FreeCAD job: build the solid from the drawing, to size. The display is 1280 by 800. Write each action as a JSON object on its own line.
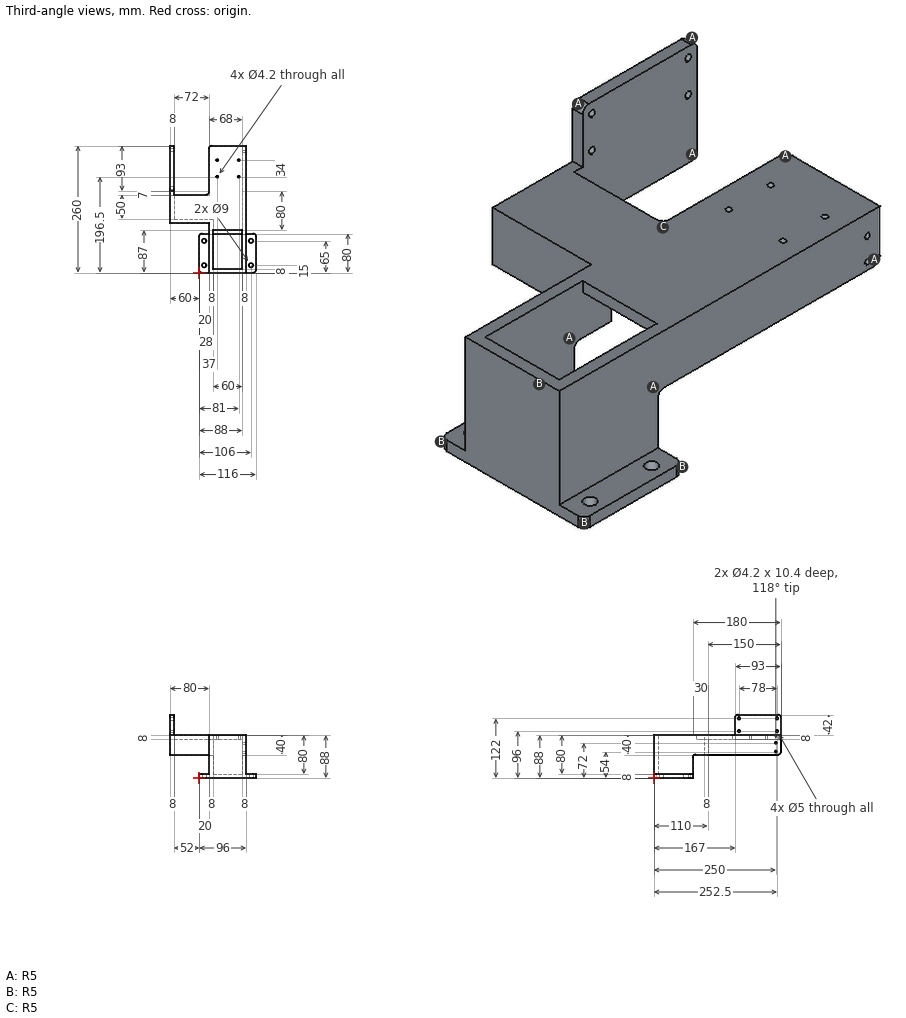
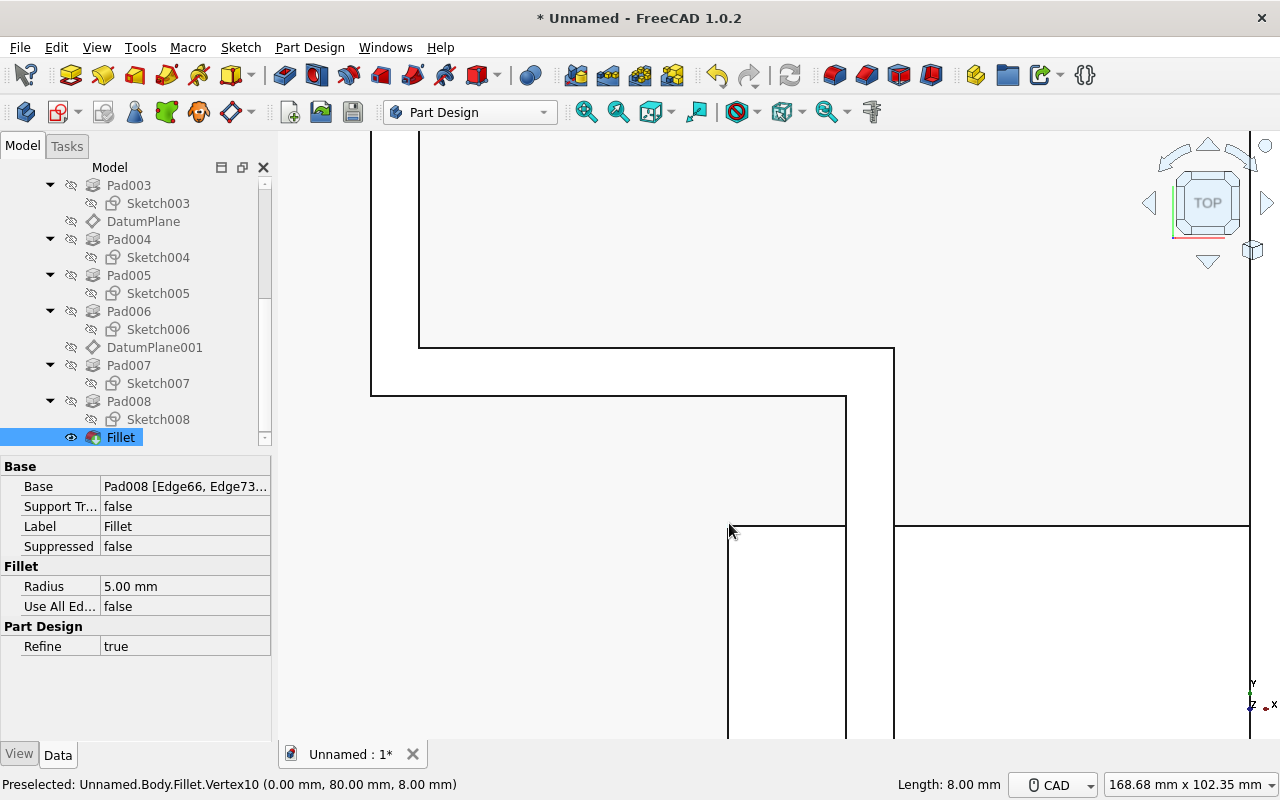
{"action": "left_click", "coordinate": [588, 112]}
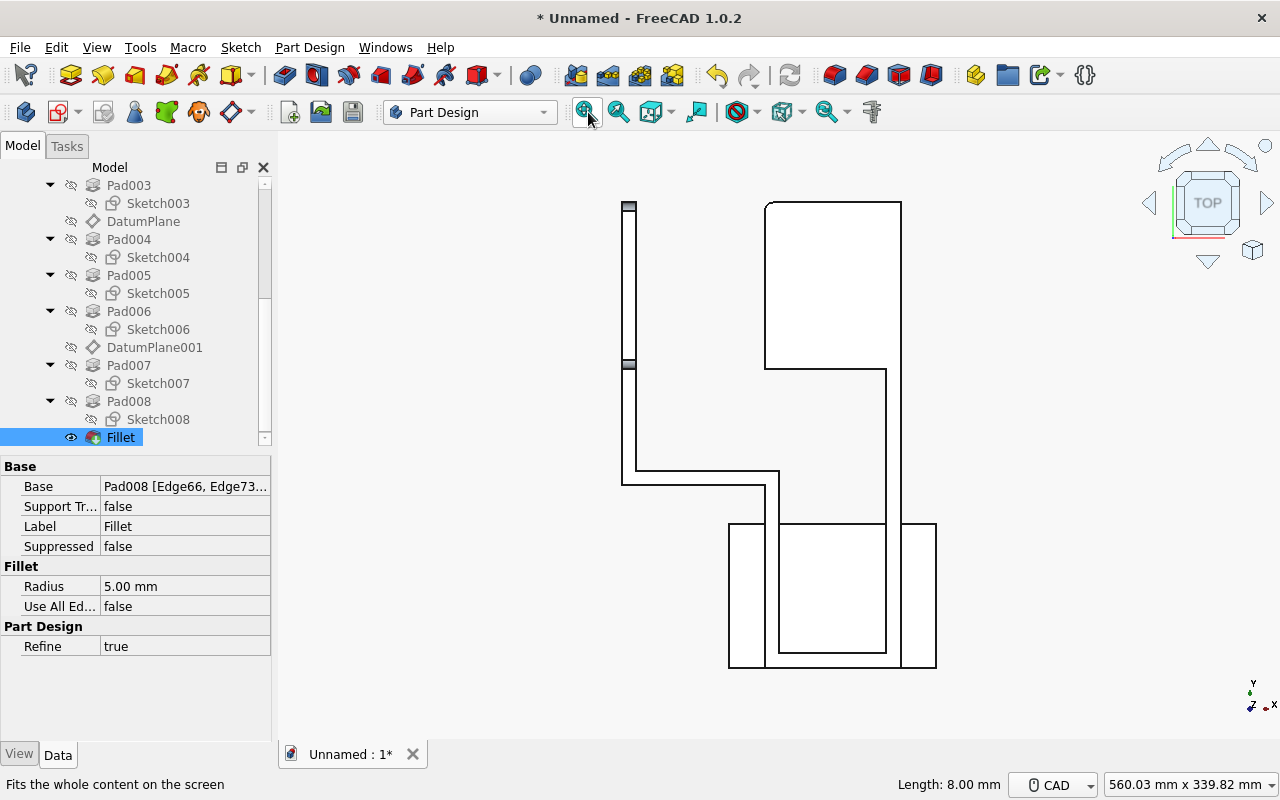
{"action": "key", "text": "0"}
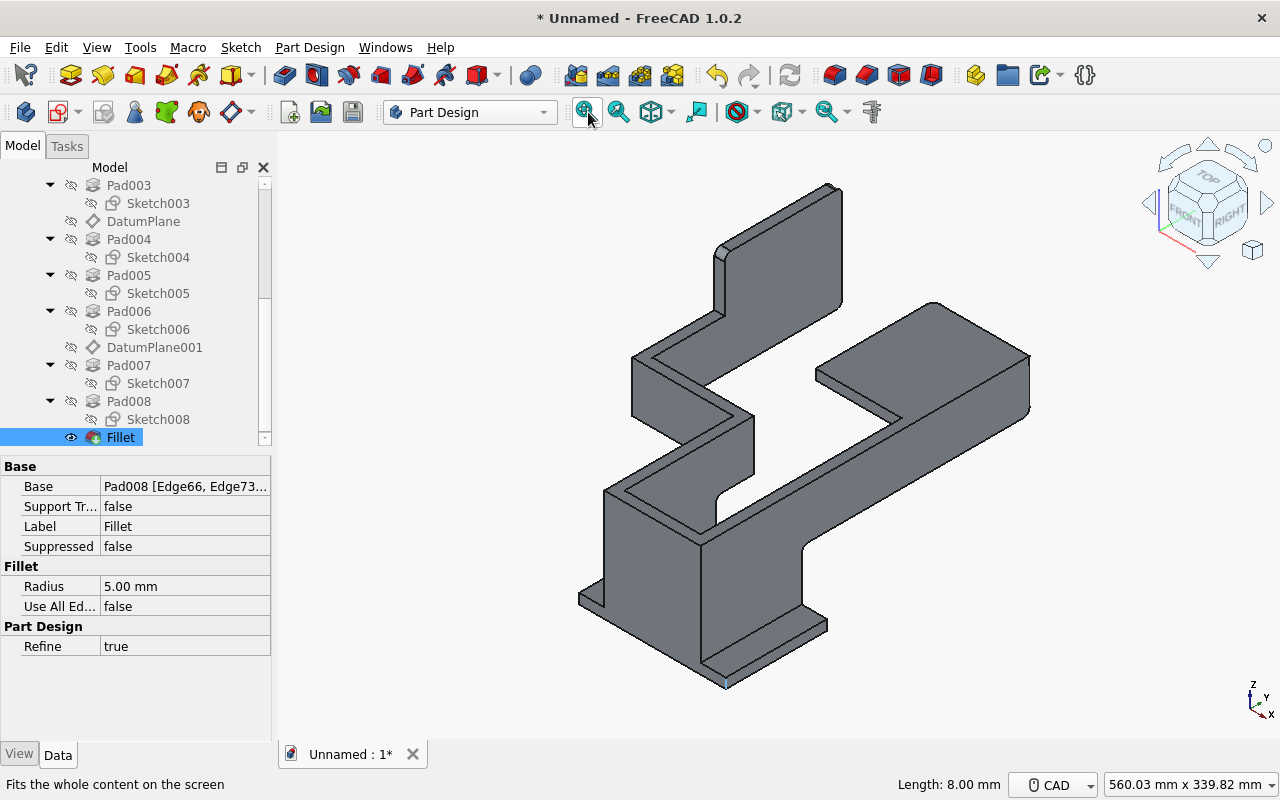
{"action": "scroll", "coordinate": [680, 539], "scroll_direction": "up", "scroll_amount": 6}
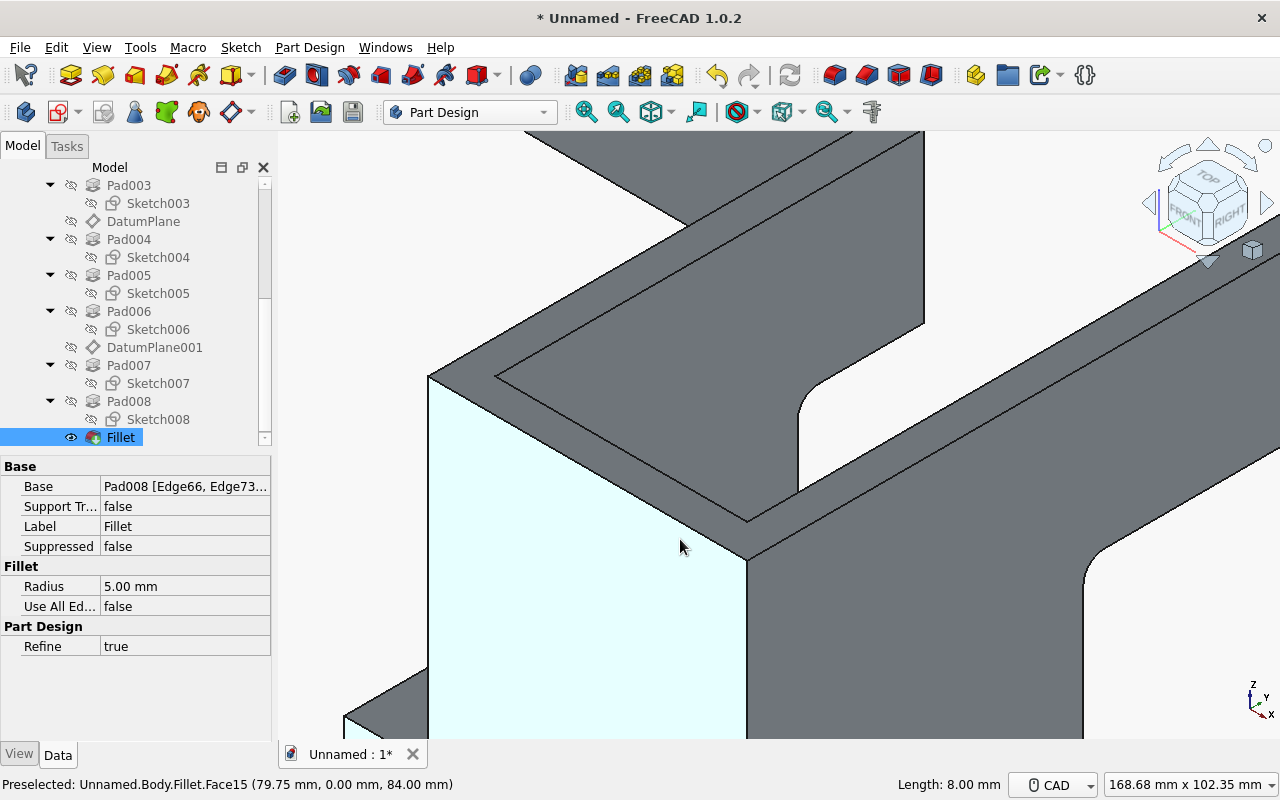
{"action": "left_click", "coordinate": [588, 112]}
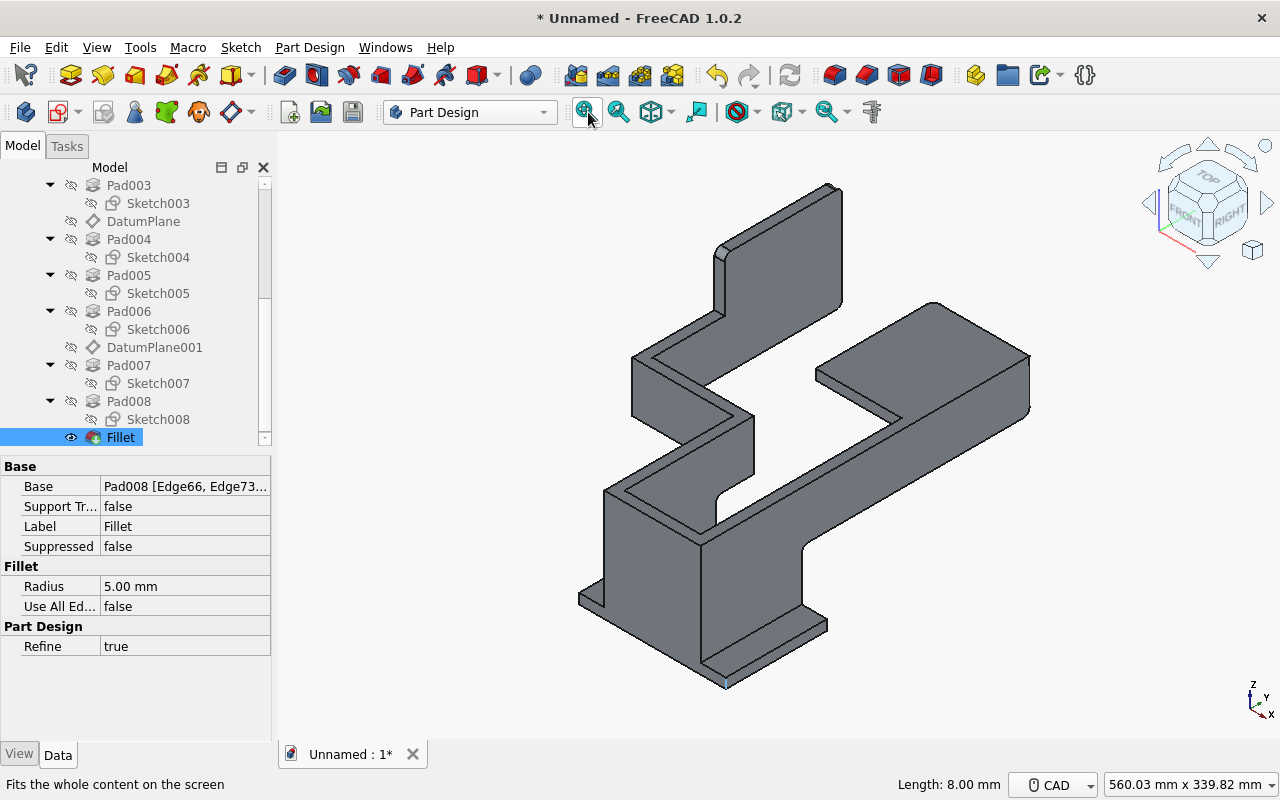
{"action": "key", "text": "1"}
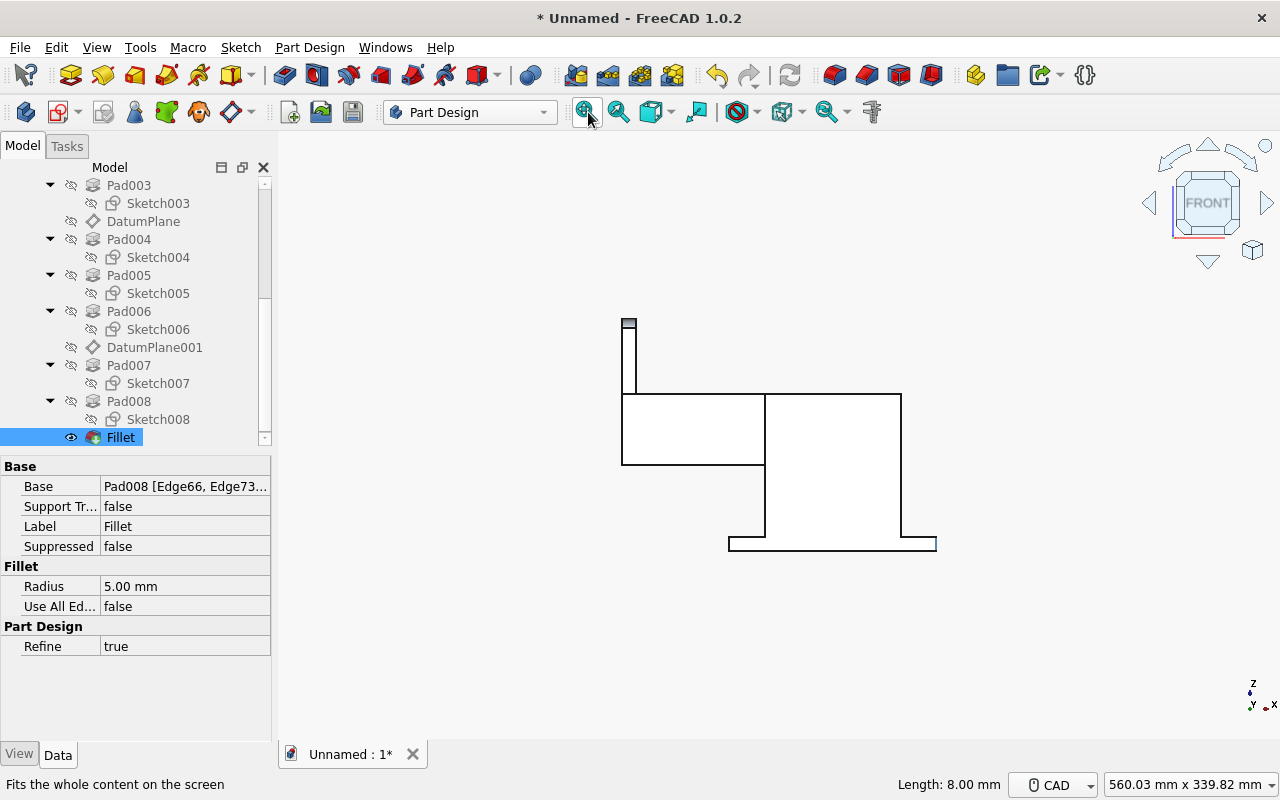
{"action": "left_click", "coordinate": [588, 112]}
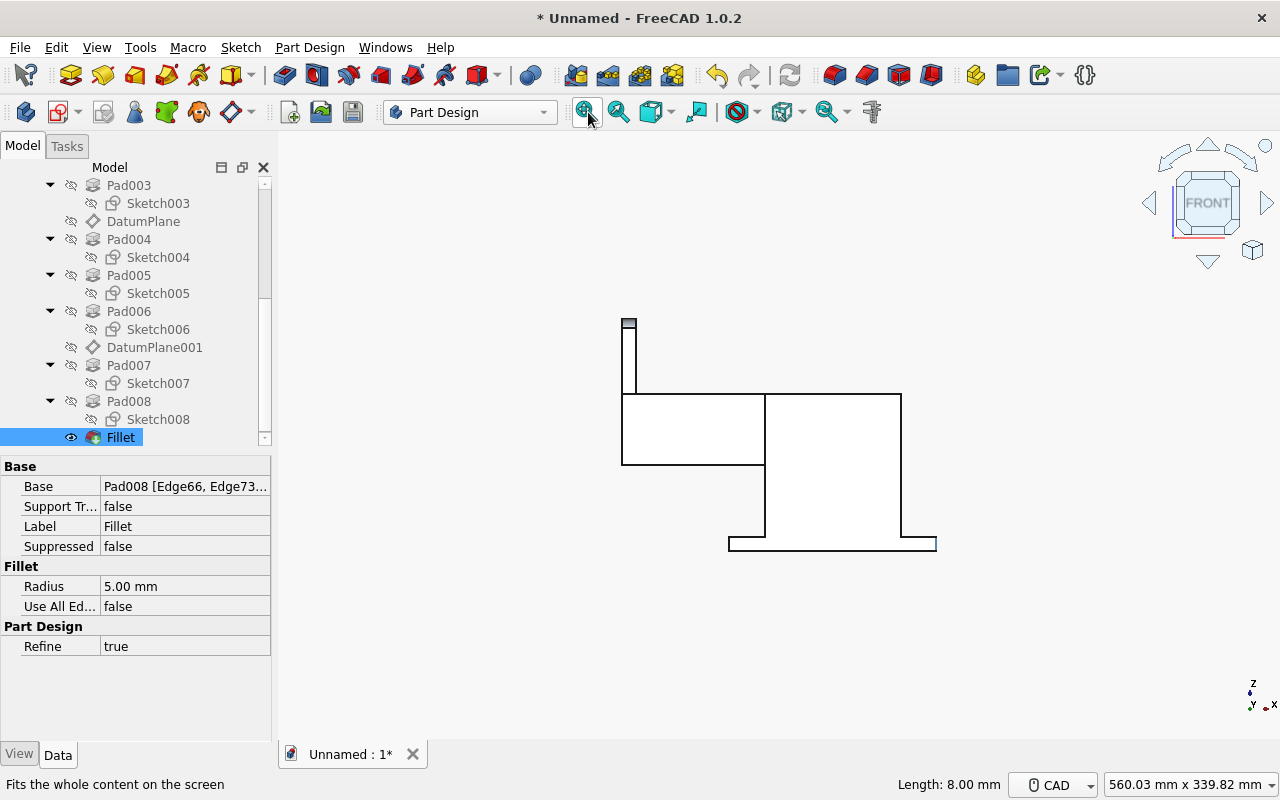
{"action": "left_click", "coordinate": [729, 543], "text": "ctrl"}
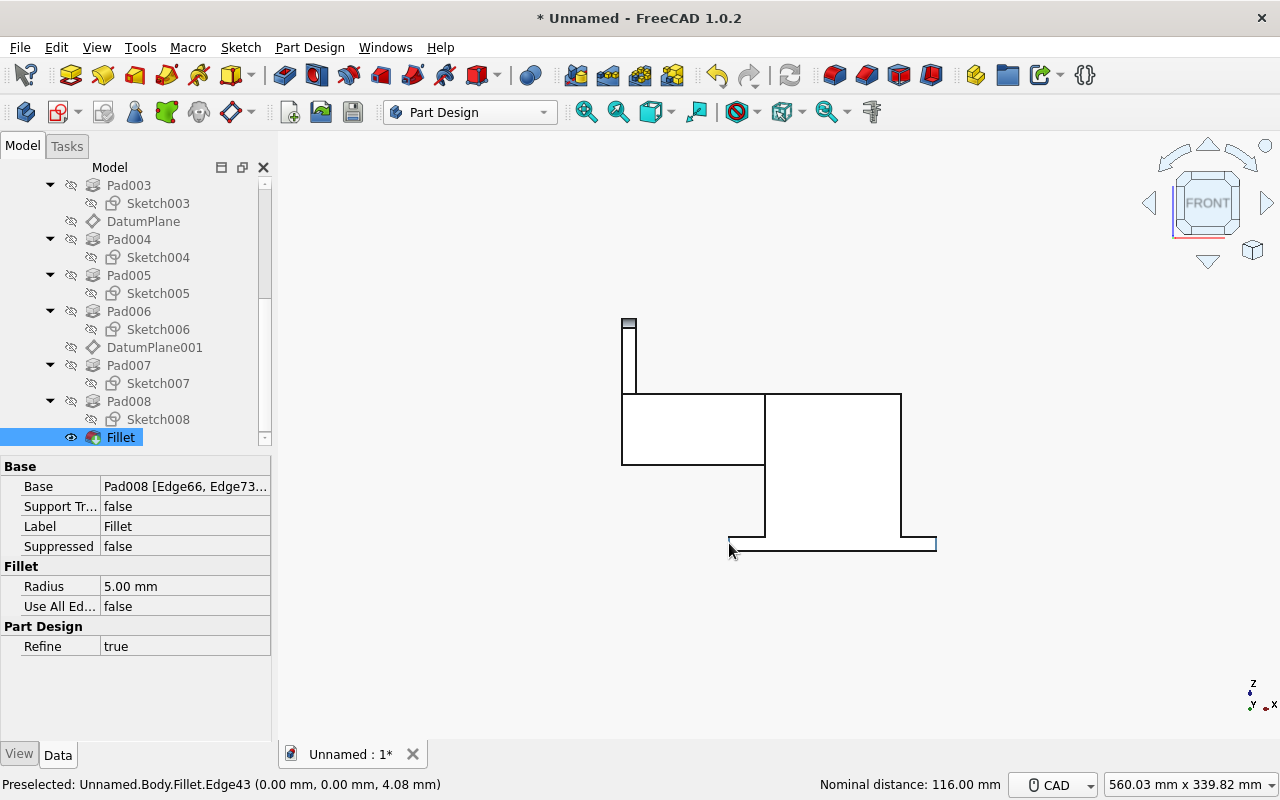
{"action": "scroll", "coordinate": [729, 543], "scroll_direction": "up", "scroll_amount": 6}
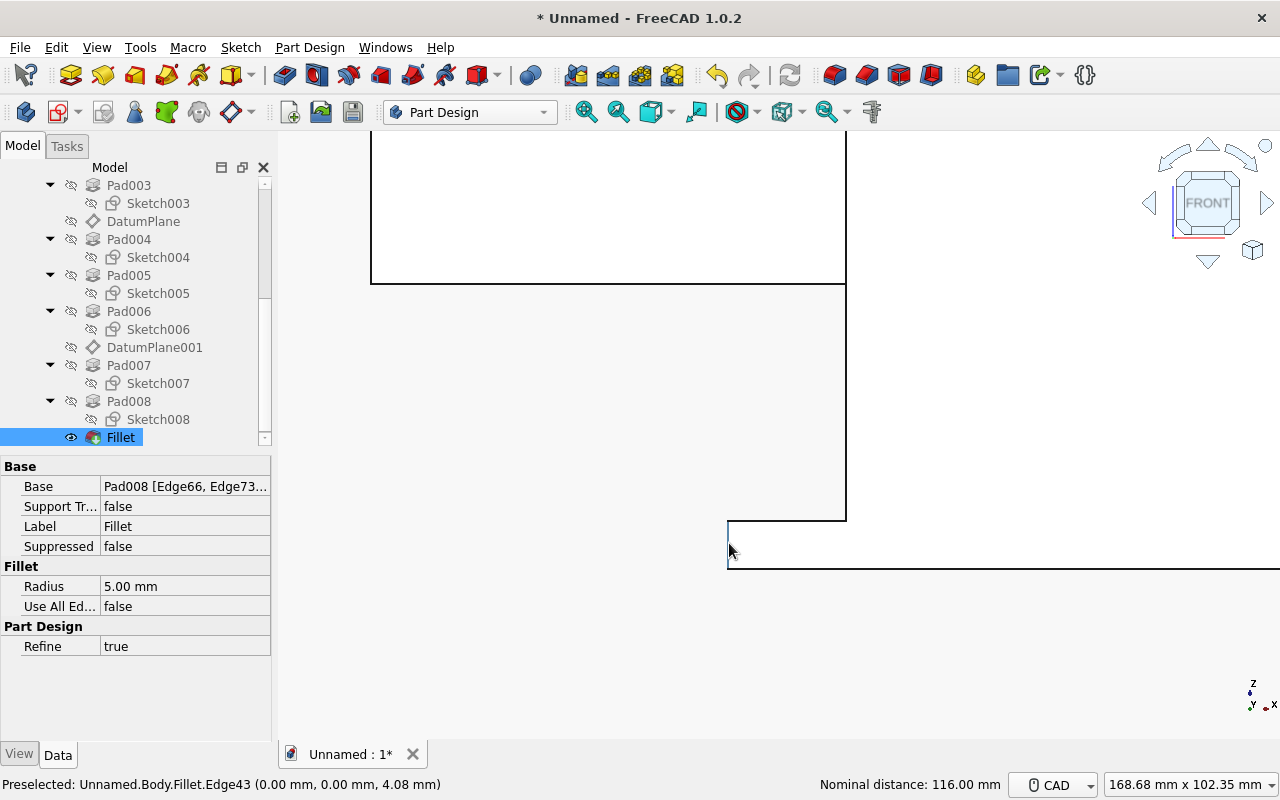
{"action": "left_click", "coordinate": [588, 112]}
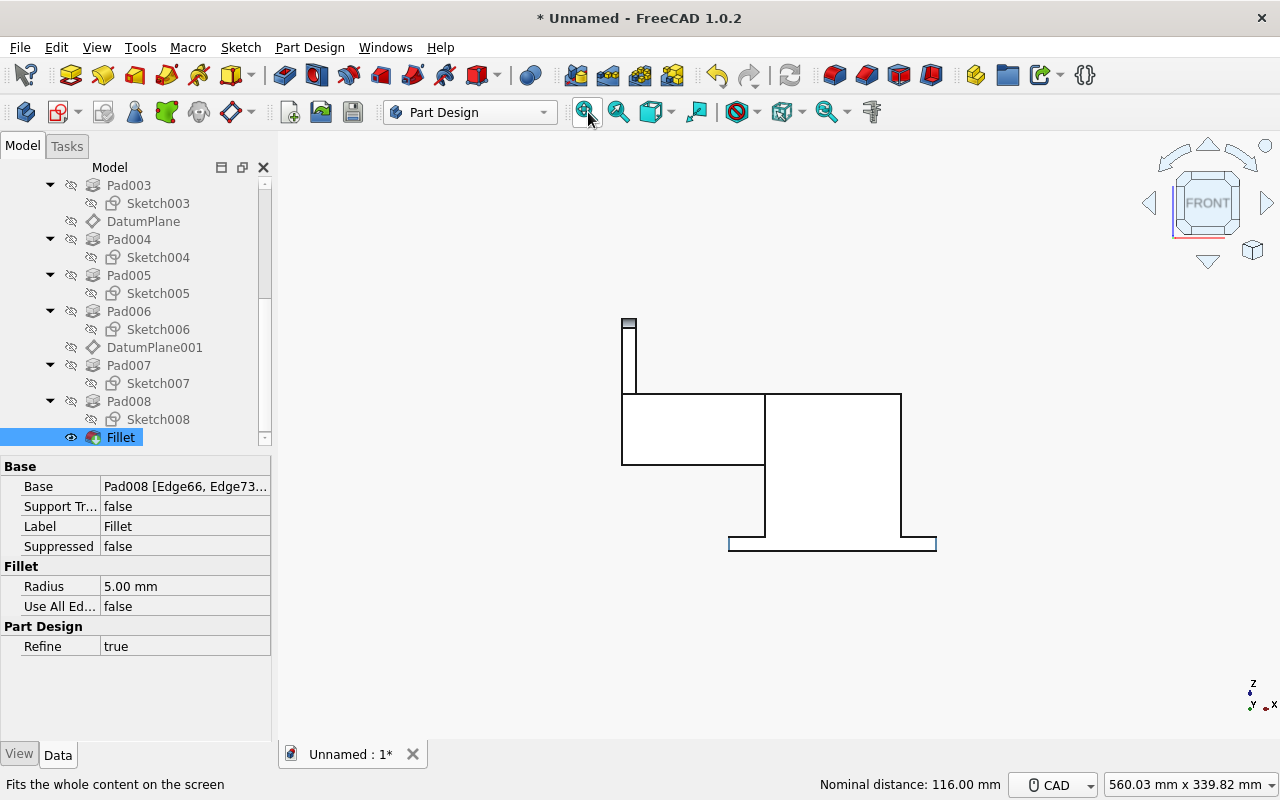
{"action": "key", "text": "3"}